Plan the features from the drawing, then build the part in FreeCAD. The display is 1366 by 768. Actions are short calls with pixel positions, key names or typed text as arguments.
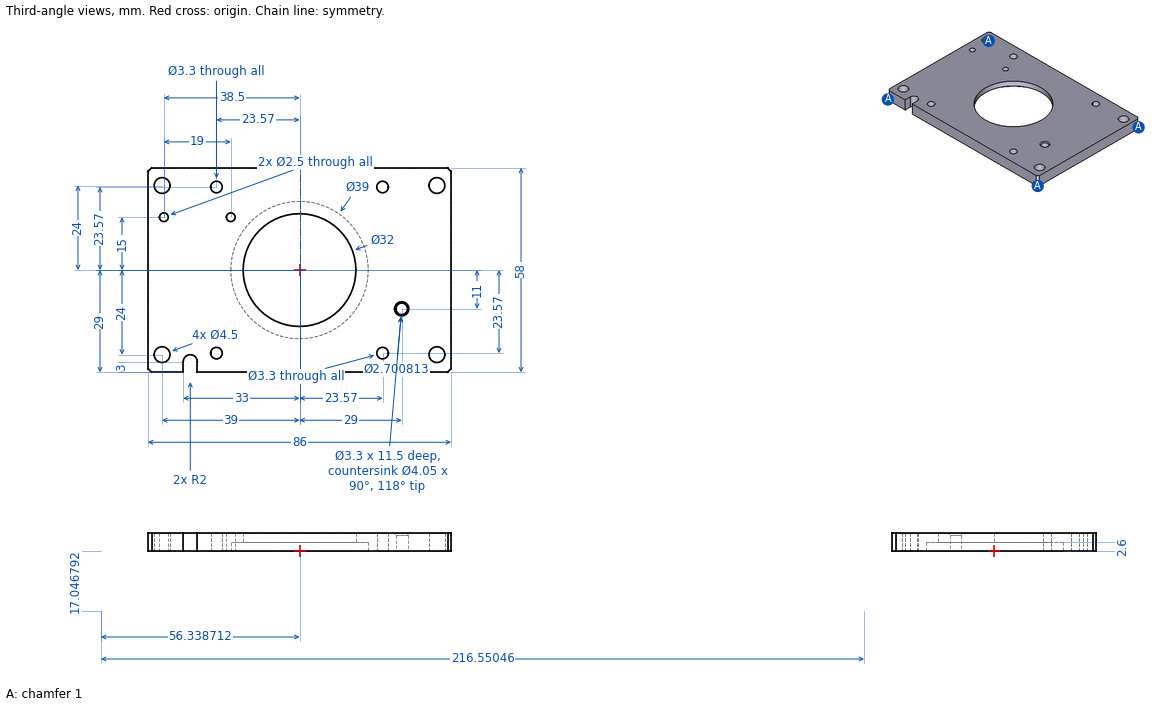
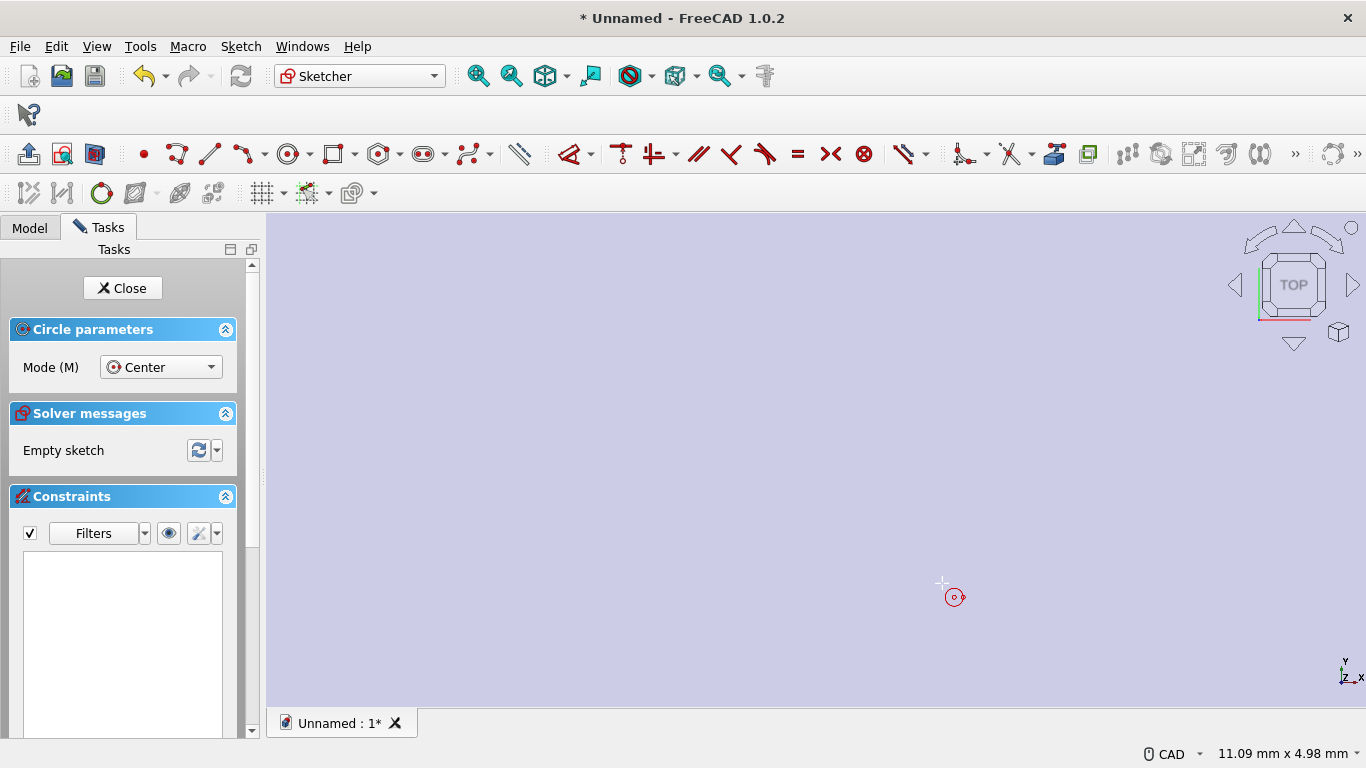
click(738, 437)
move(854, 321)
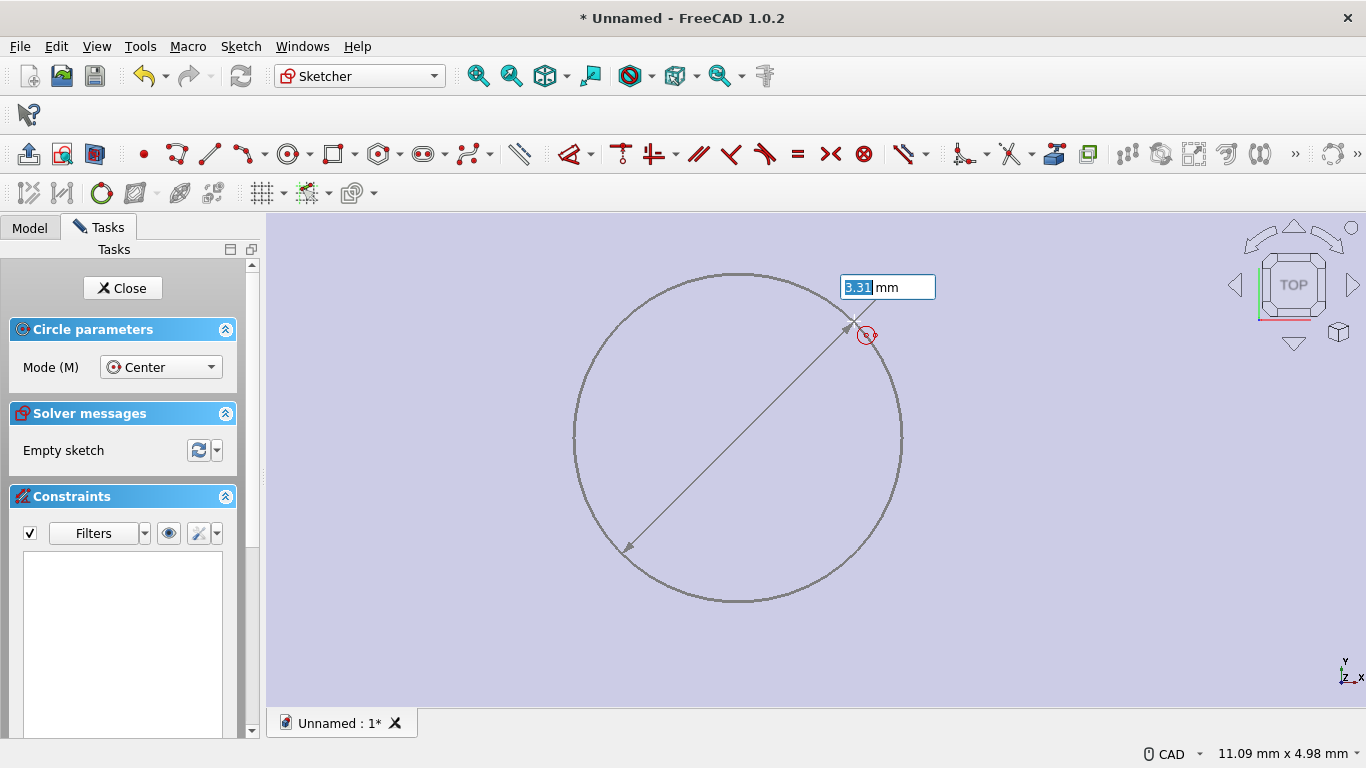
text(3.3)
key(Return)
key(Escape)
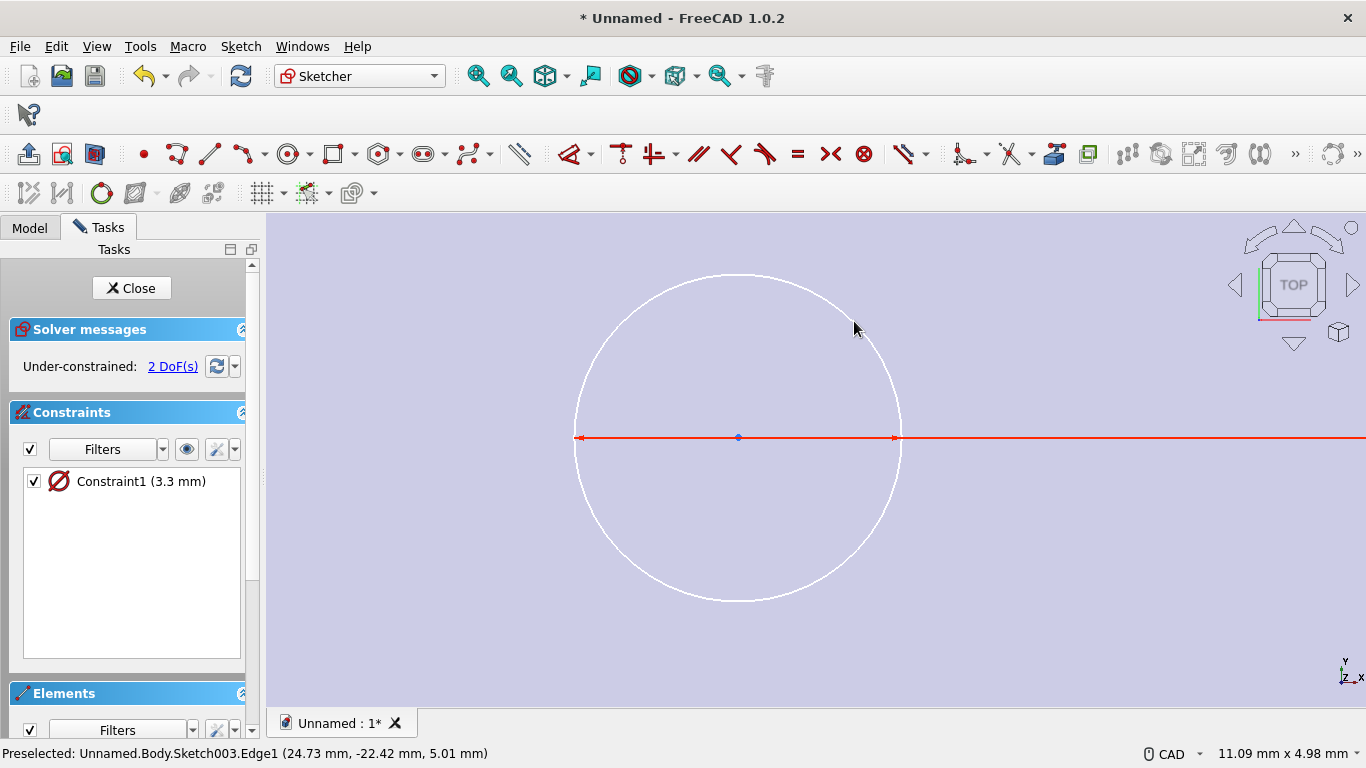
key(d)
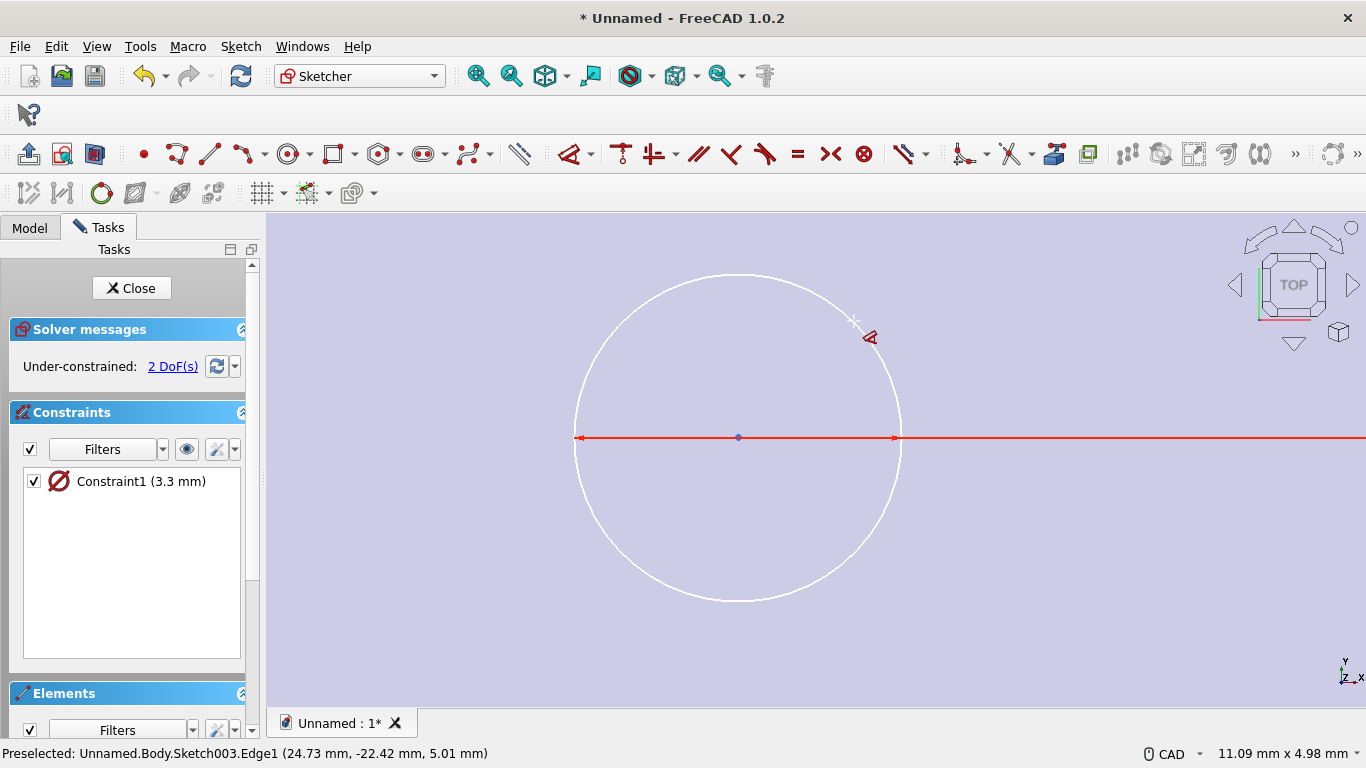
click(738, 438)
click(516, 472)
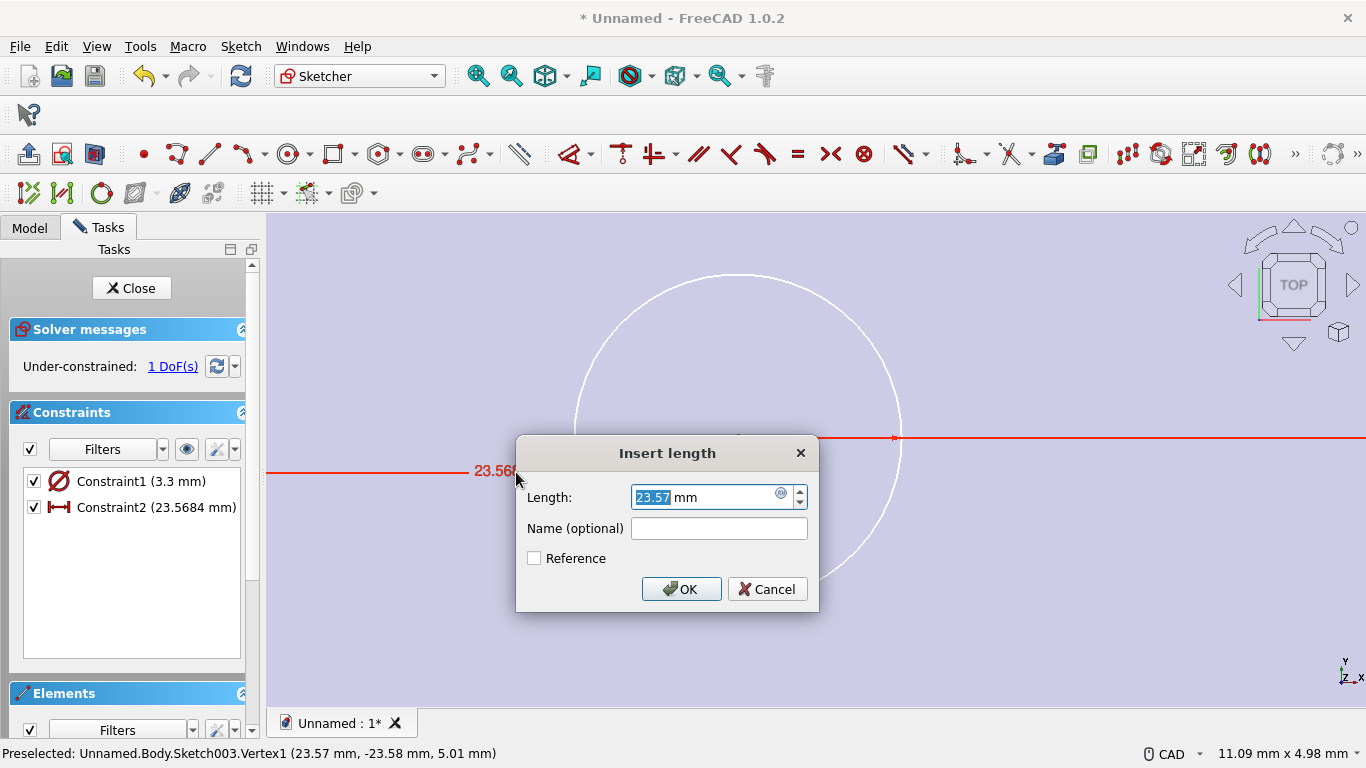
text(23.57)
key(Return)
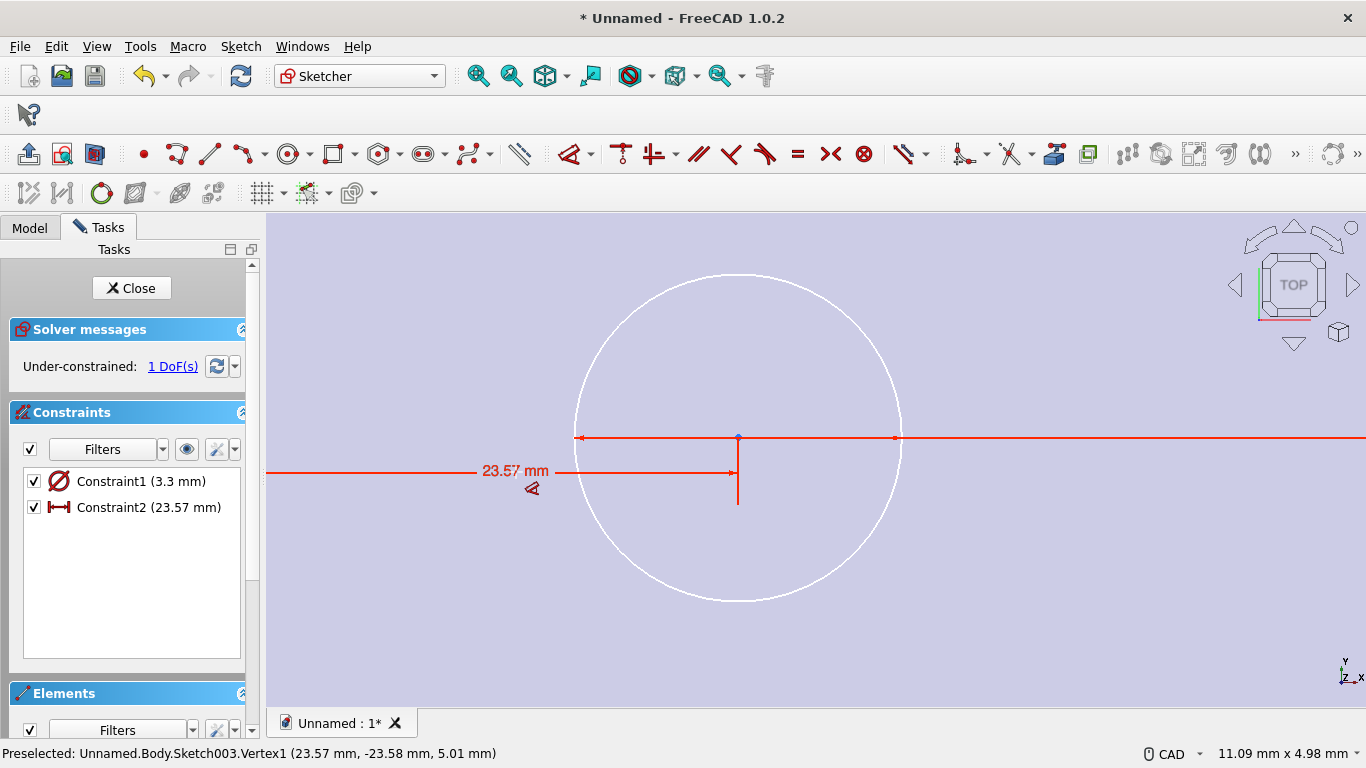
click(738, 438)
click(772, 340)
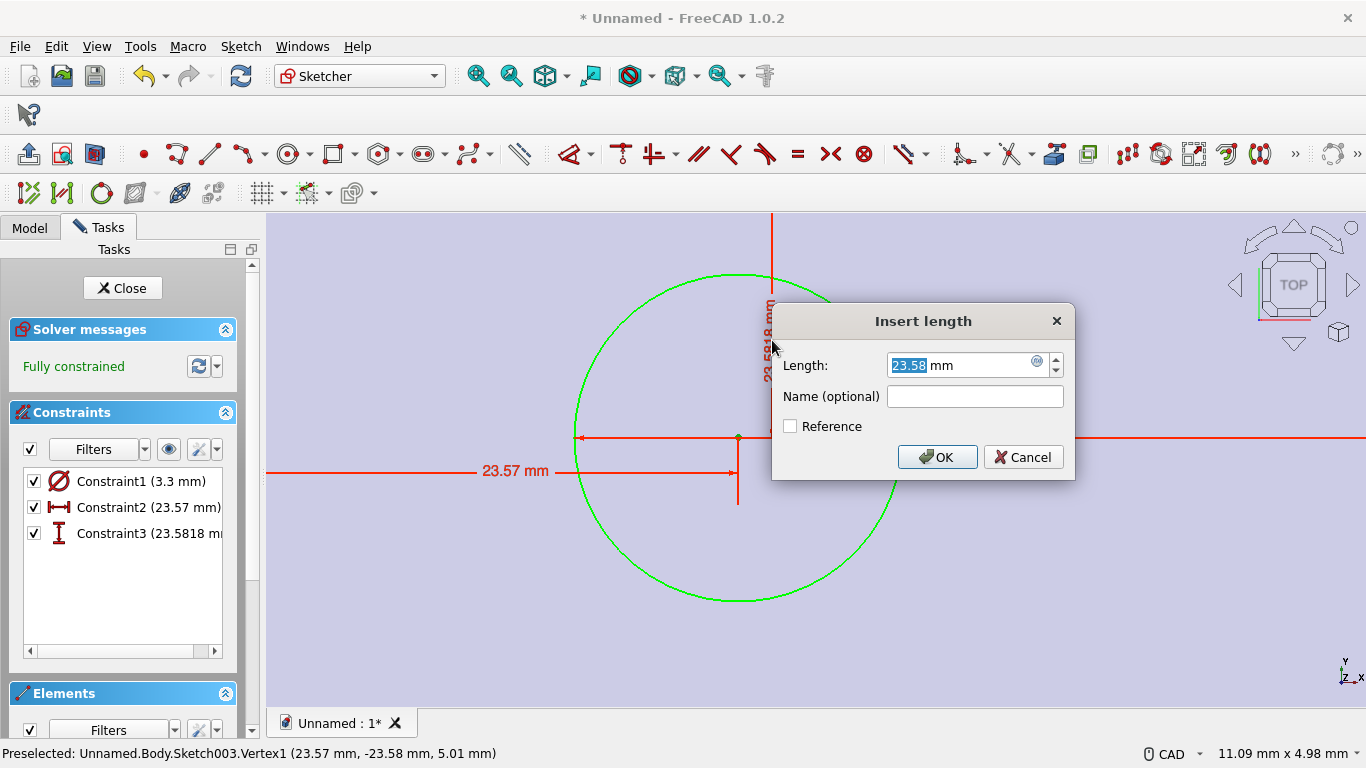
text(23.57)
key(Return)
key(Escape)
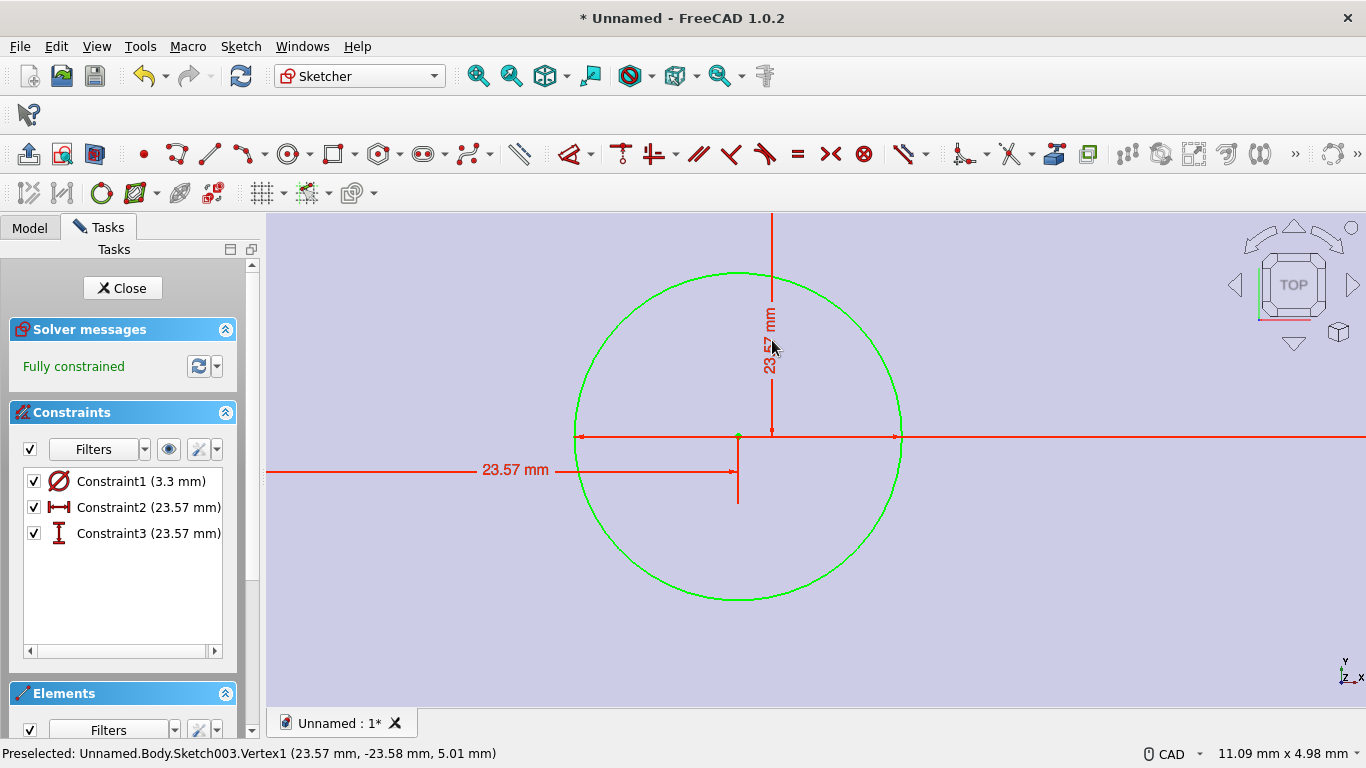
click(123, 288)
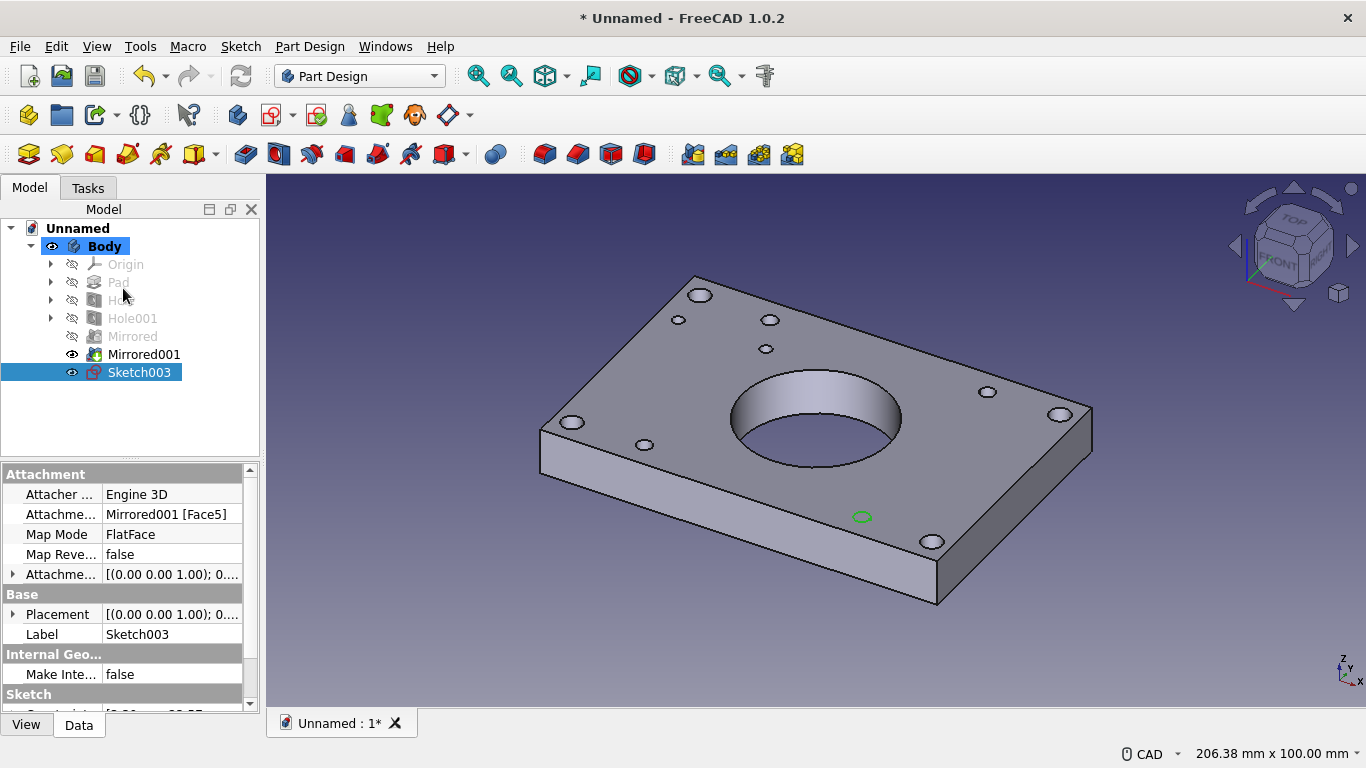
click(279, 154)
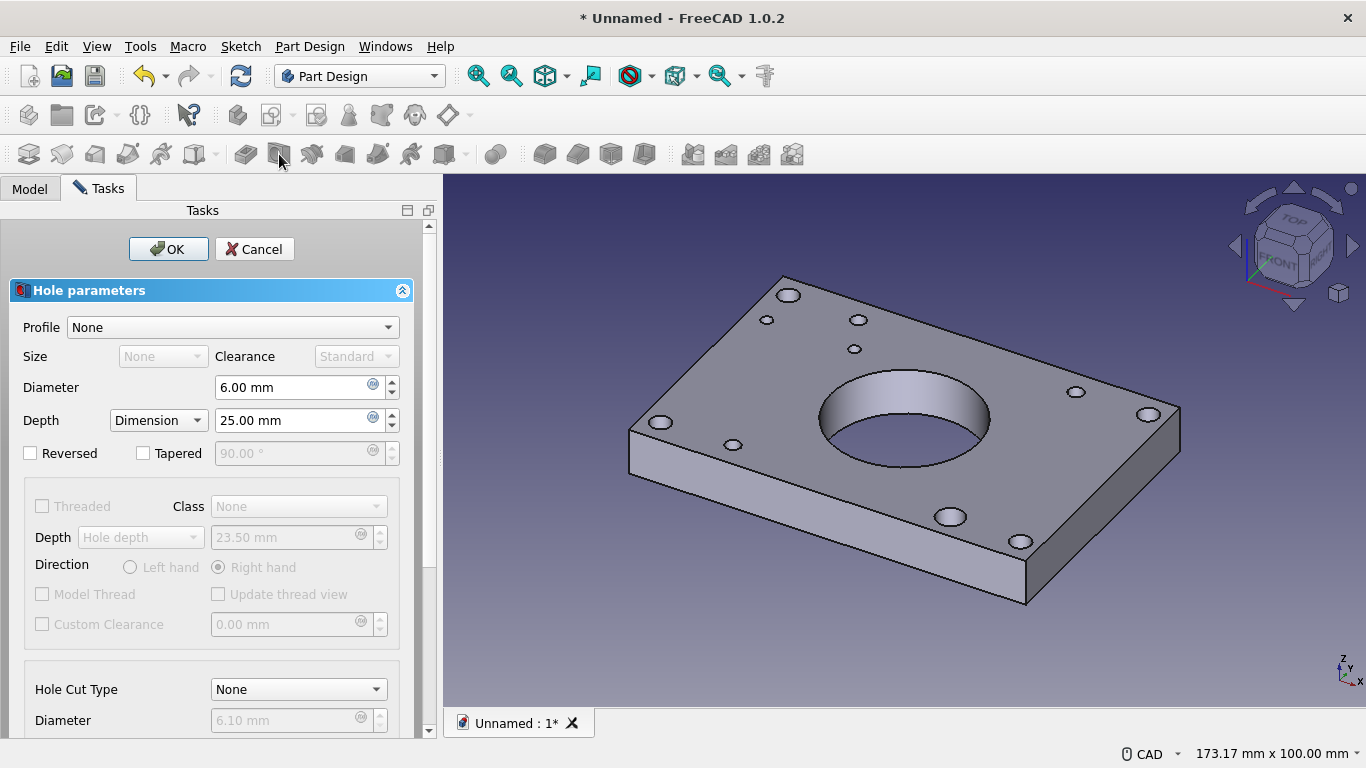
triple_click(300, 388)